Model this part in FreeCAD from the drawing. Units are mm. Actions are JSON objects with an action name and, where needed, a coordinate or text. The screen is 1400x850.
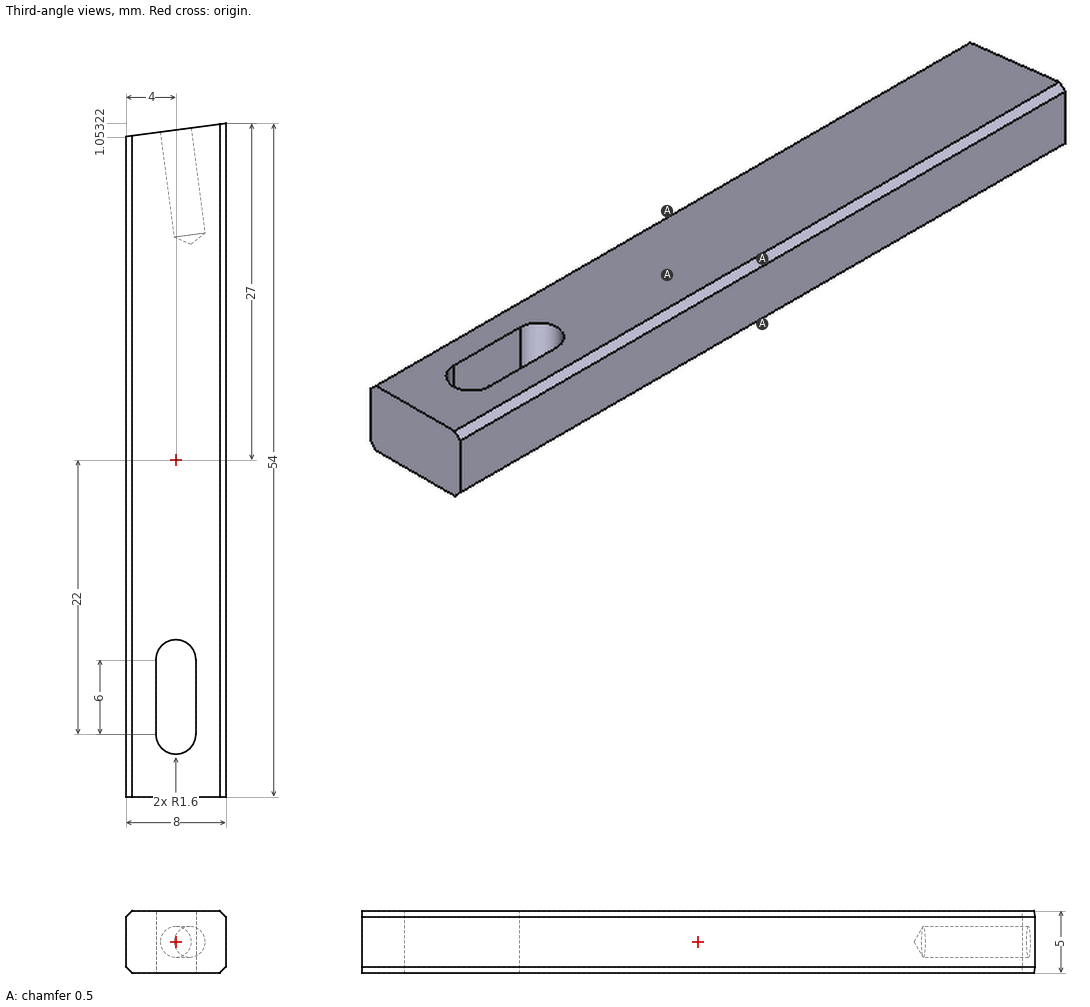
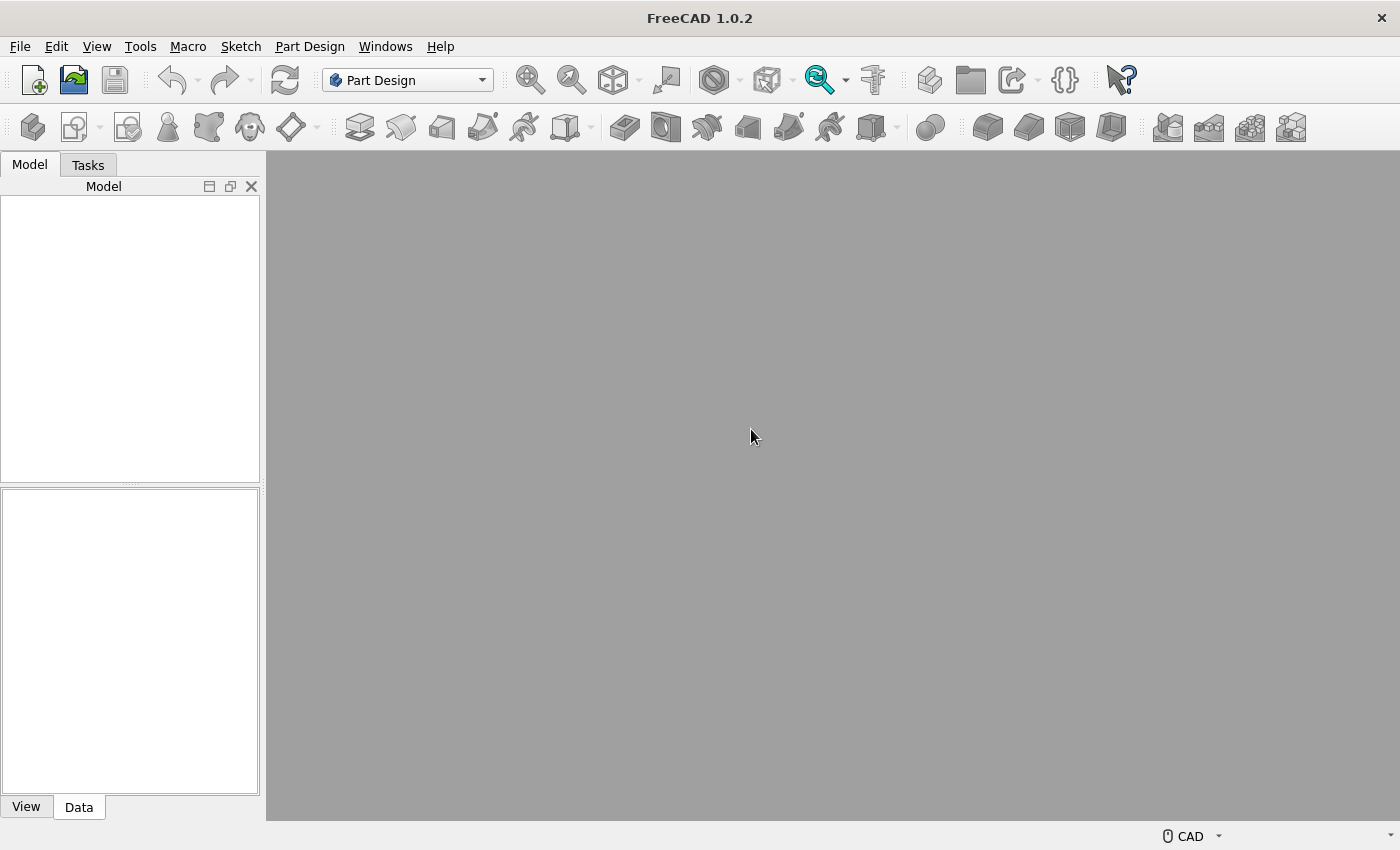
{"action": "key", "text": "ctrl+n"}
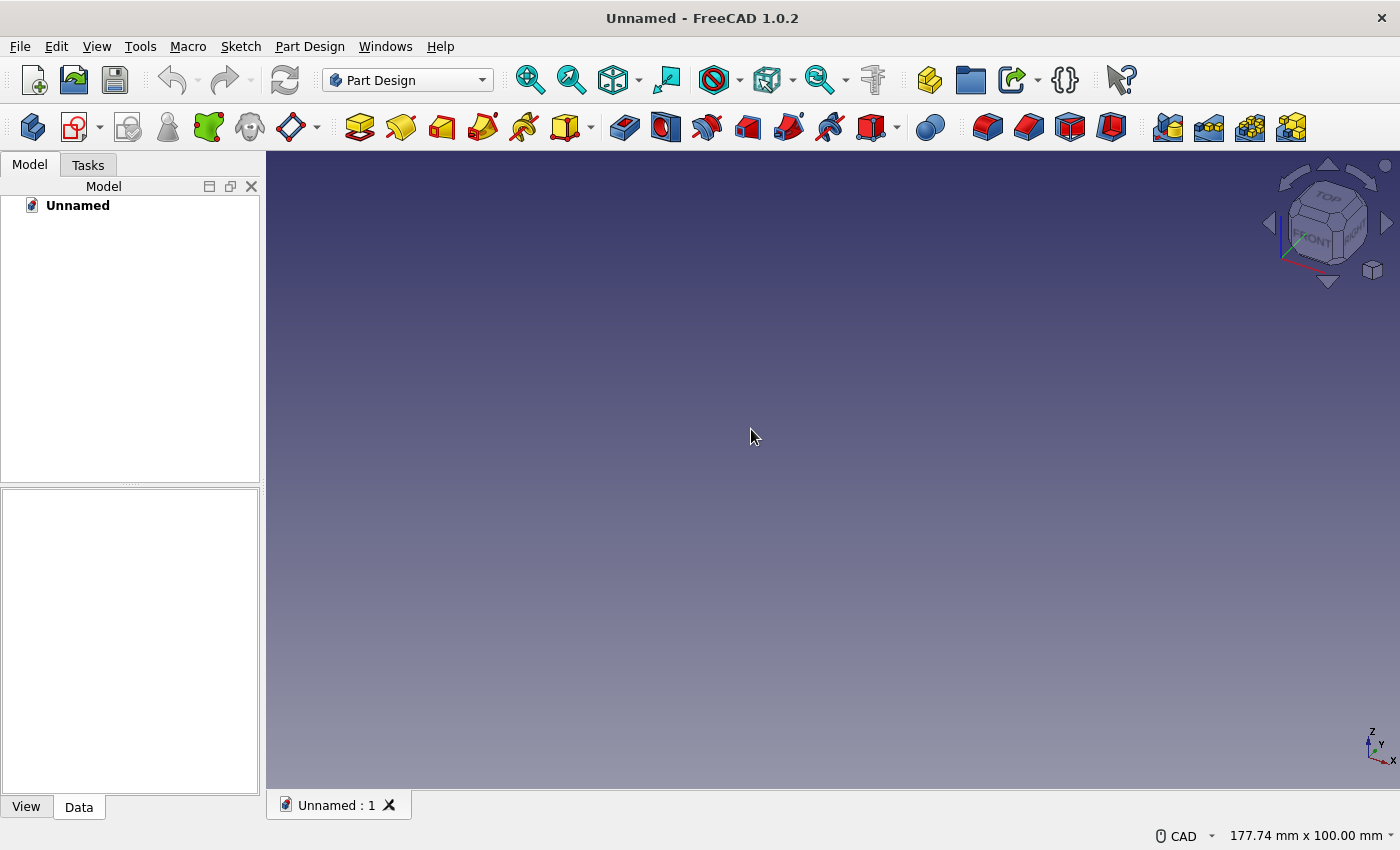
{"action": "left_click", "coordinate": [74, 128]}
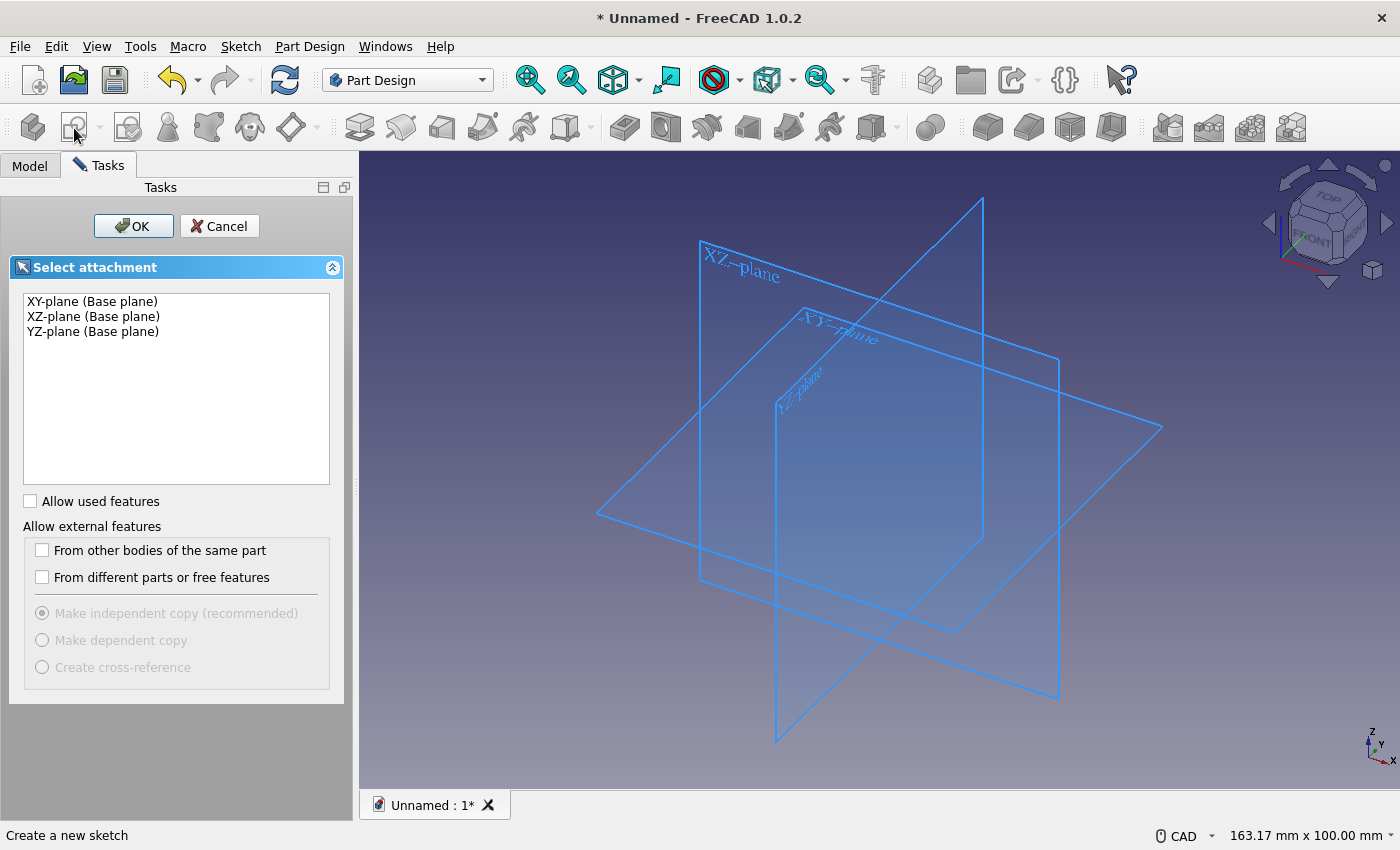
{"action": "left_click", "coordinate": [84, 302]}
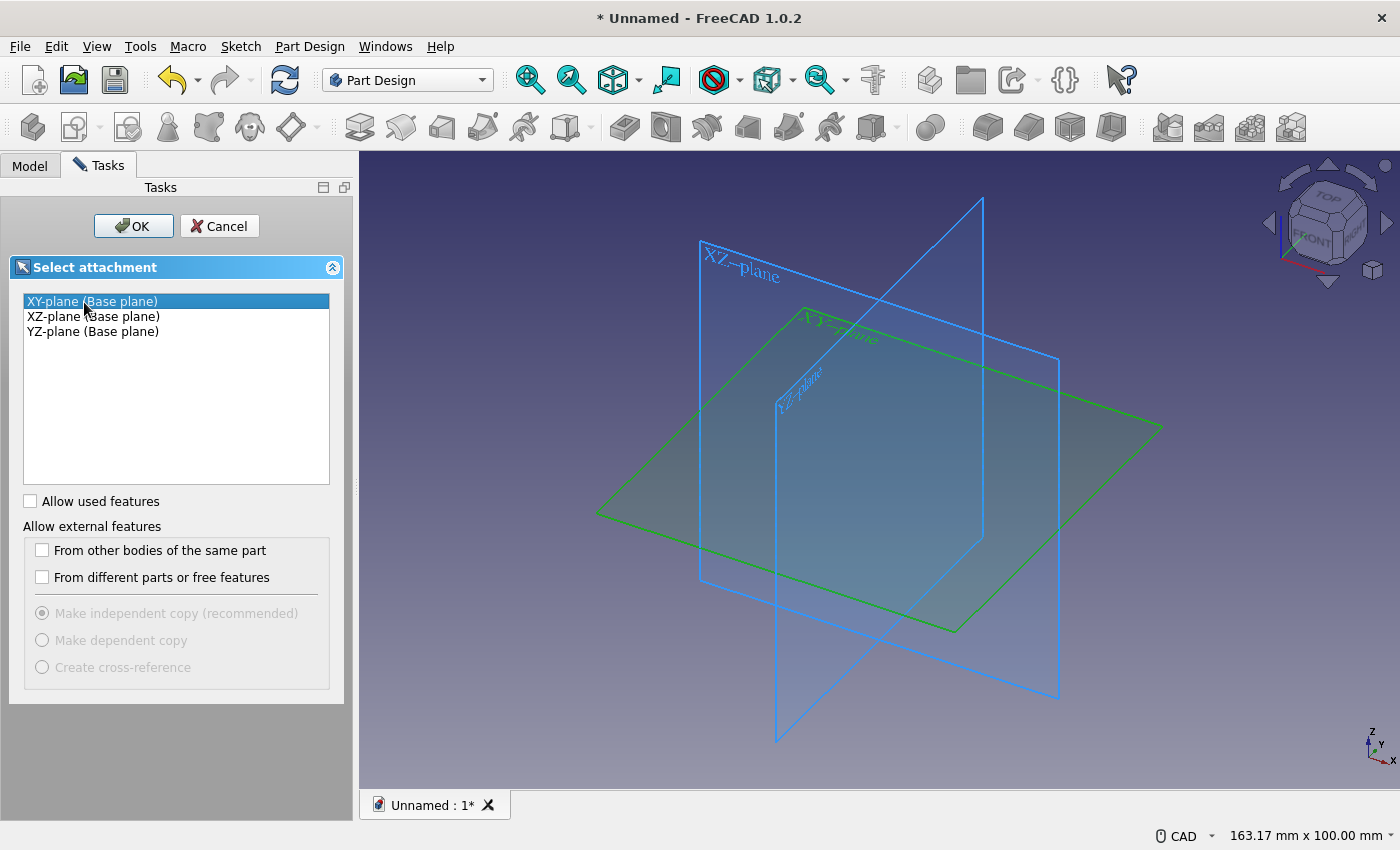
{"action": "left_click", "coordinate": [134, 226]}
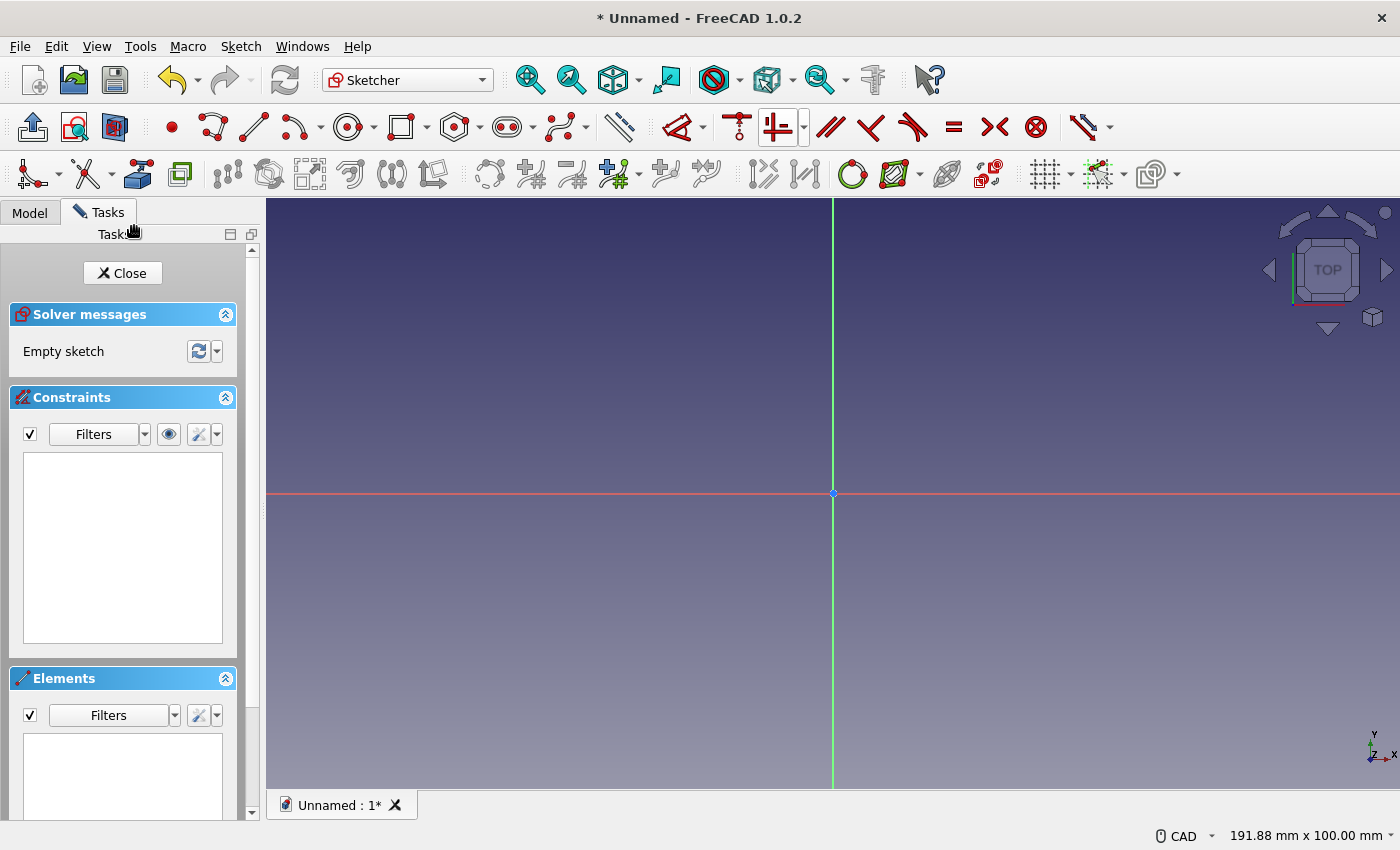
{"action": "key", "text": "g v"}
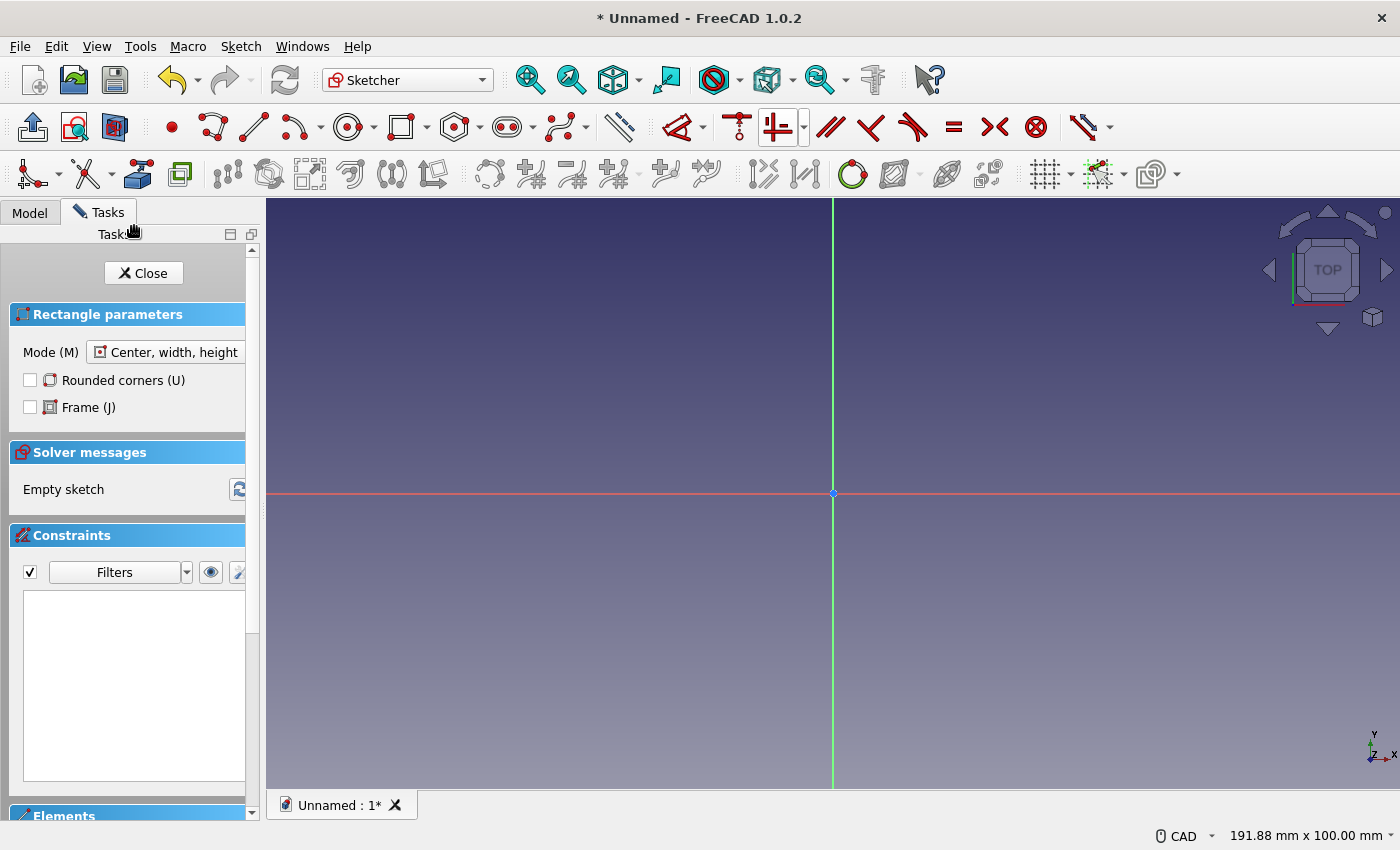
{"action": "left_click", "coordinate": [833, 494]}
{"action": "left_click", "coordinate": [857, 334]}
{"action": "key", "text": "Escape"}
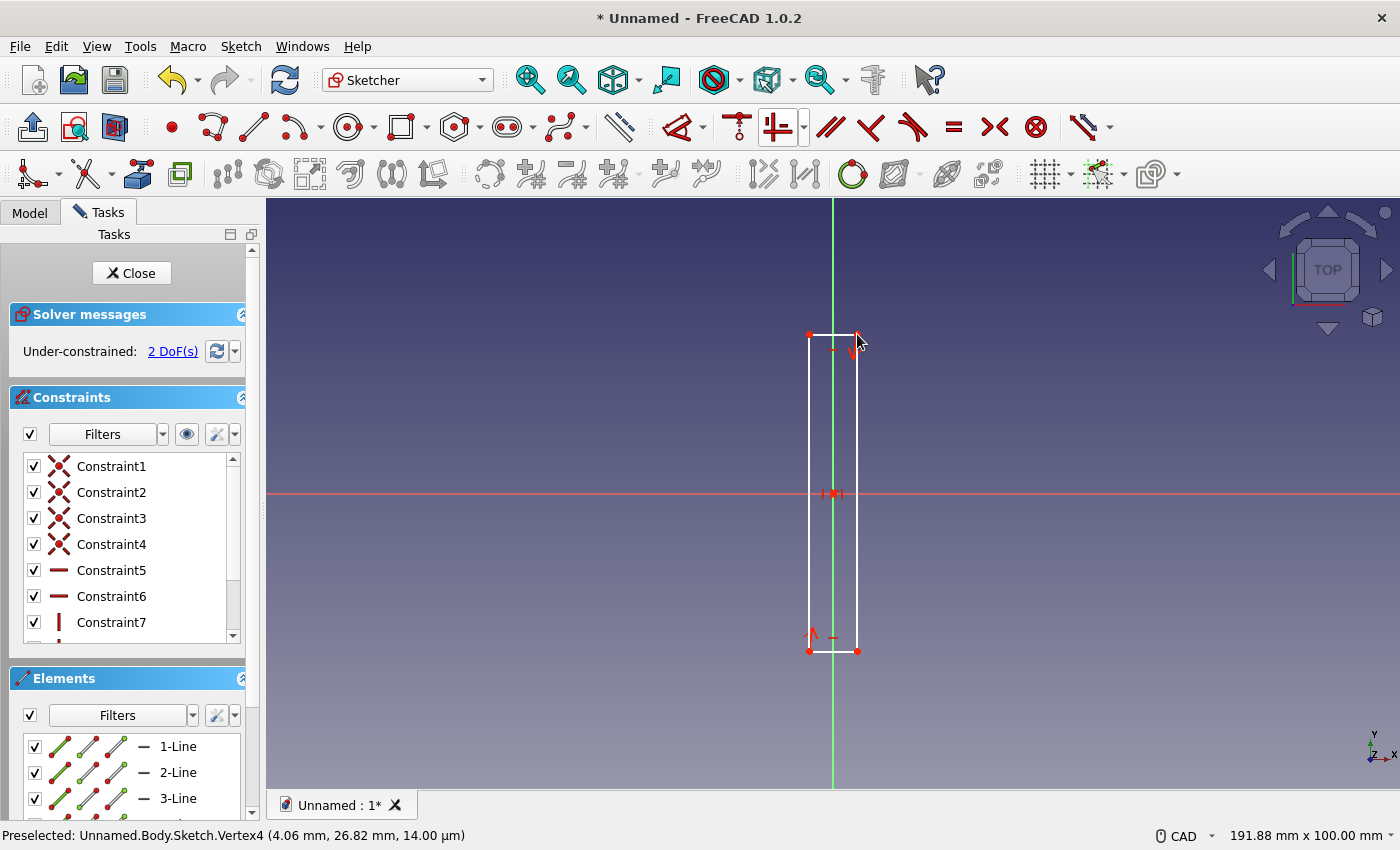
{"action": "scroll", "coordinate": [823, 652], "scroll_direction": "up", "scroll_amount": 2}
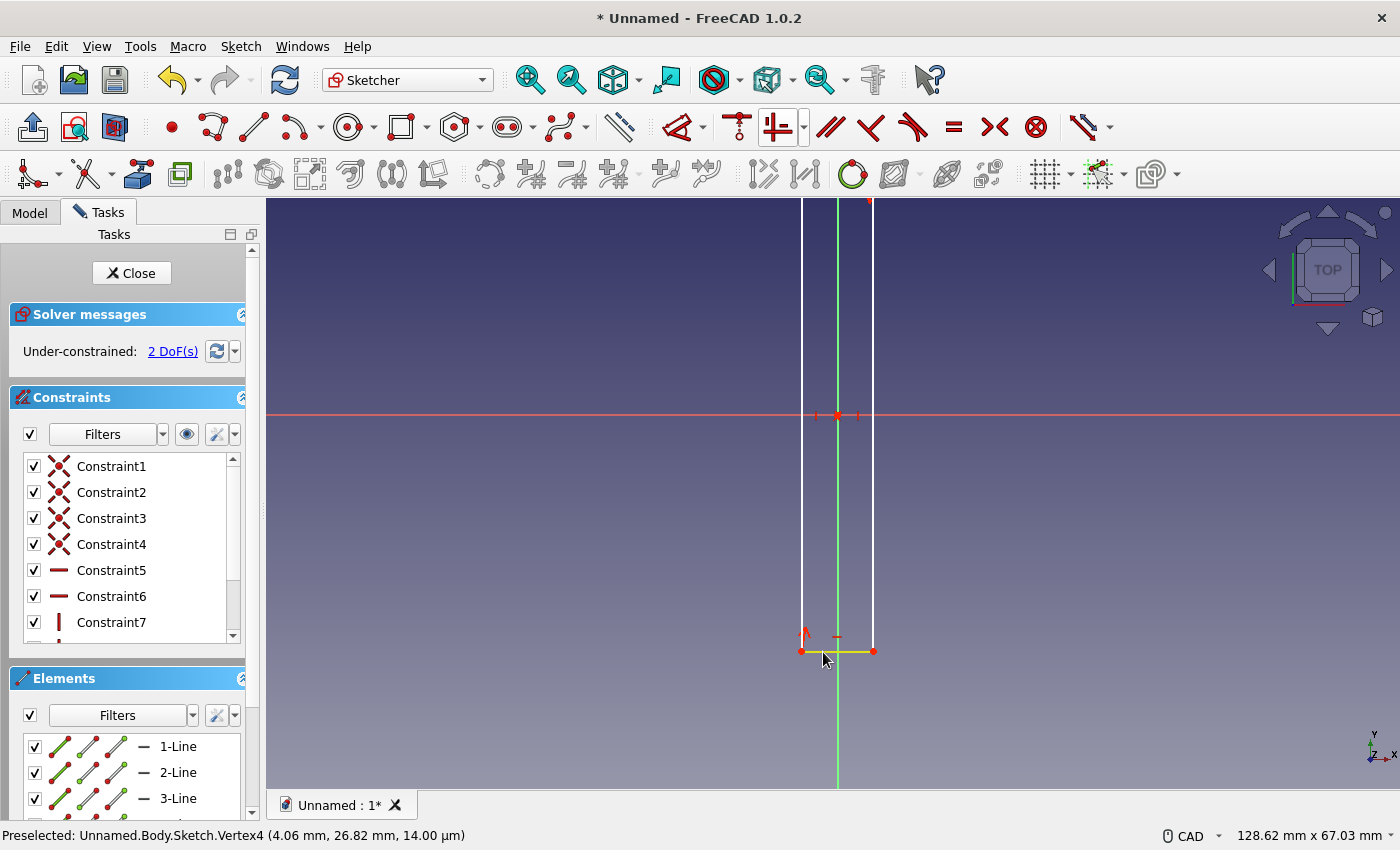
{"action": "left_click", "coordinate": [823, 652]}